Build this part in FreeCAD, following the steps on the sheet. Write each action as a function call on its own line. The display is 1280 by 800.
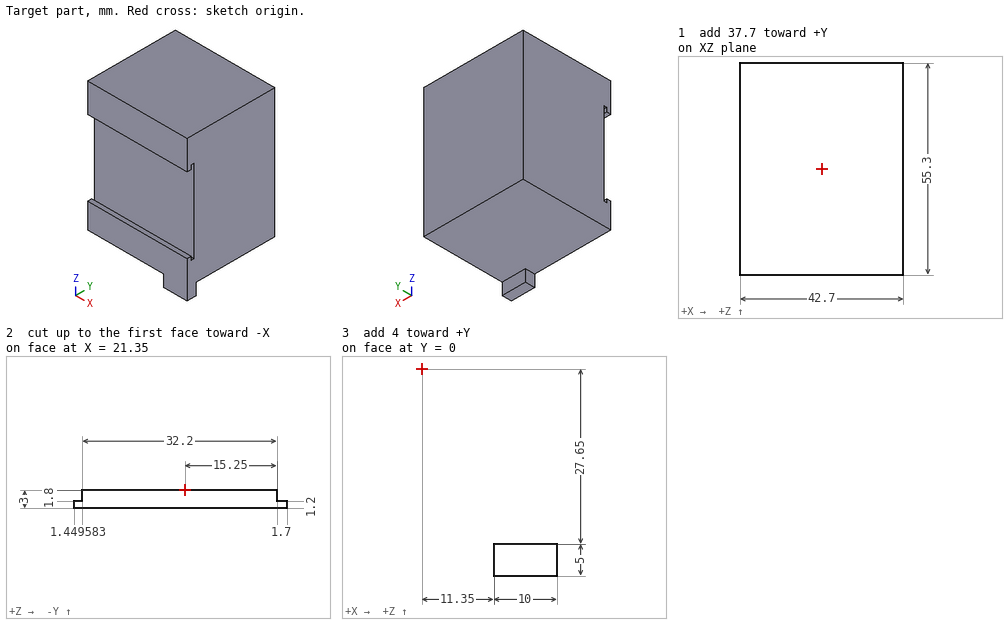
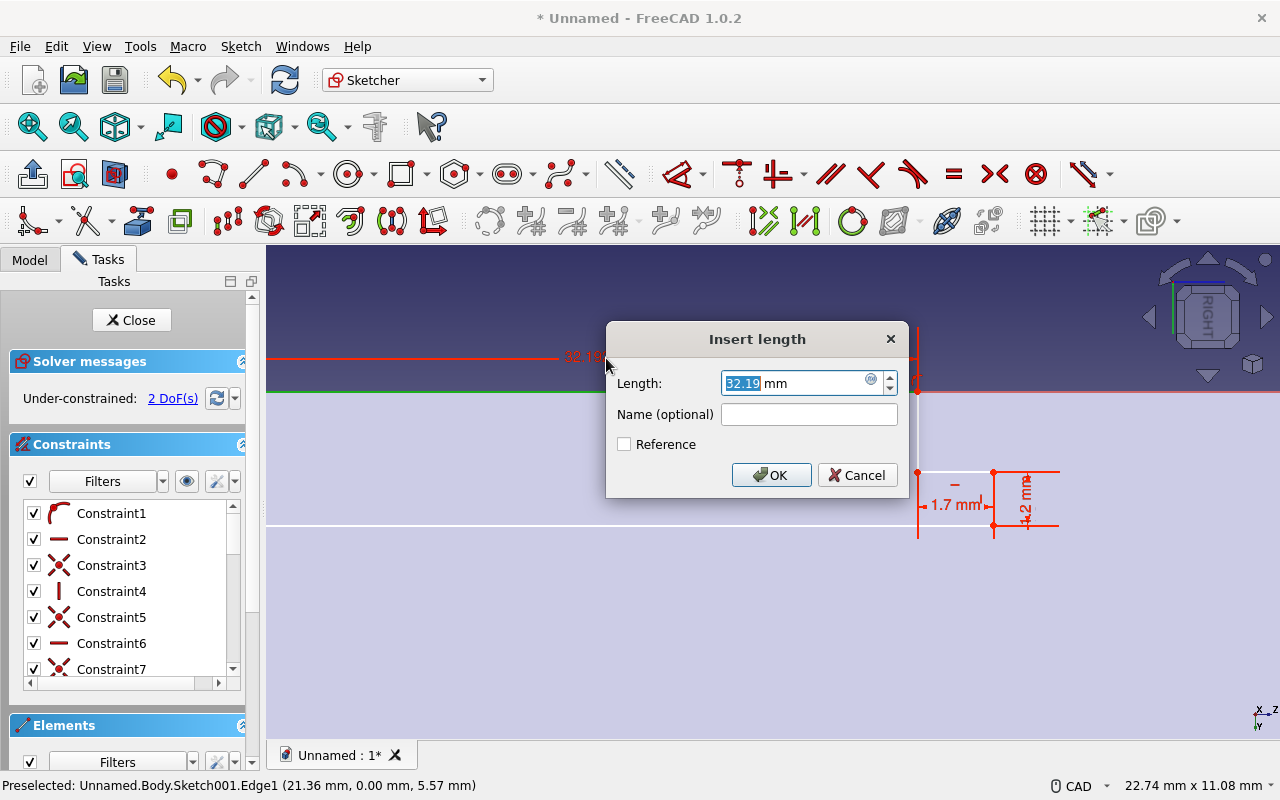
text(32.2)
key(Return)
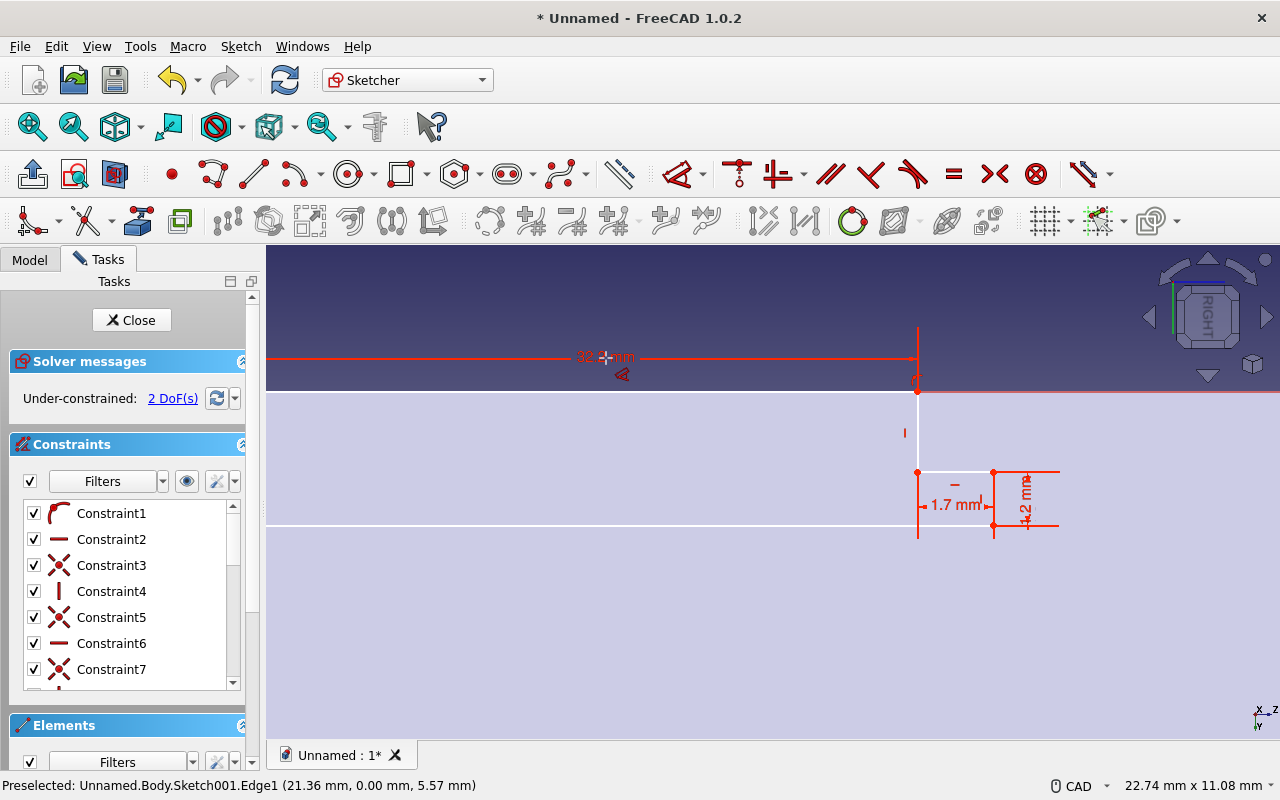
click(918, 392)
click(462, 358)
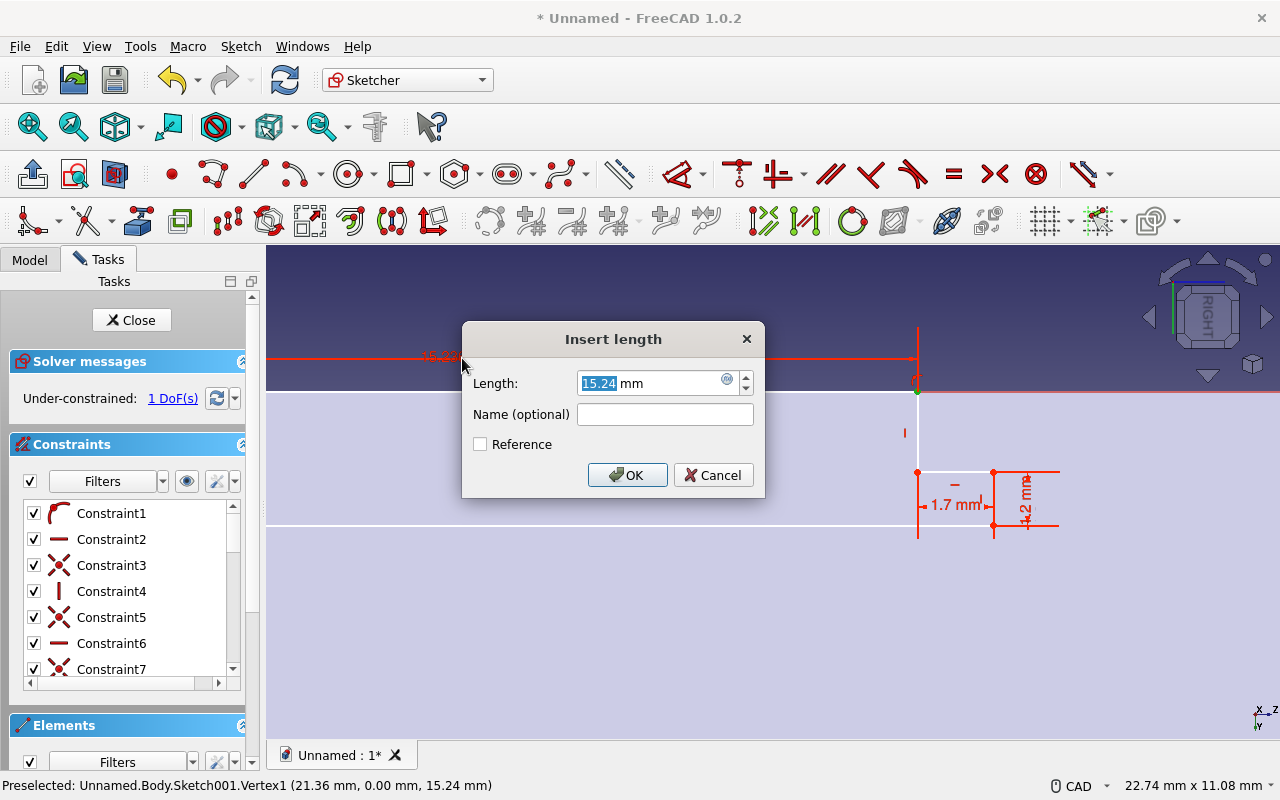
text(15.25)
key(Return)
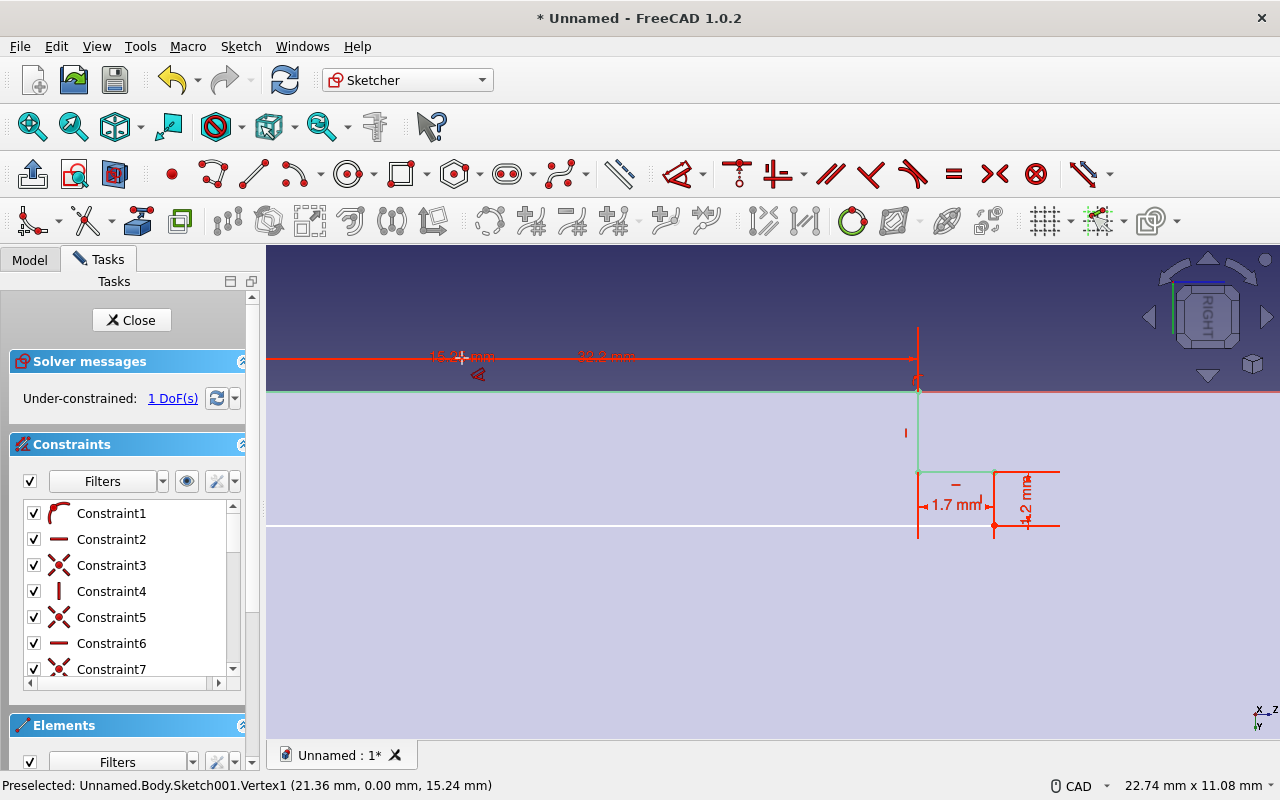
scroll(994, 511, down, 5)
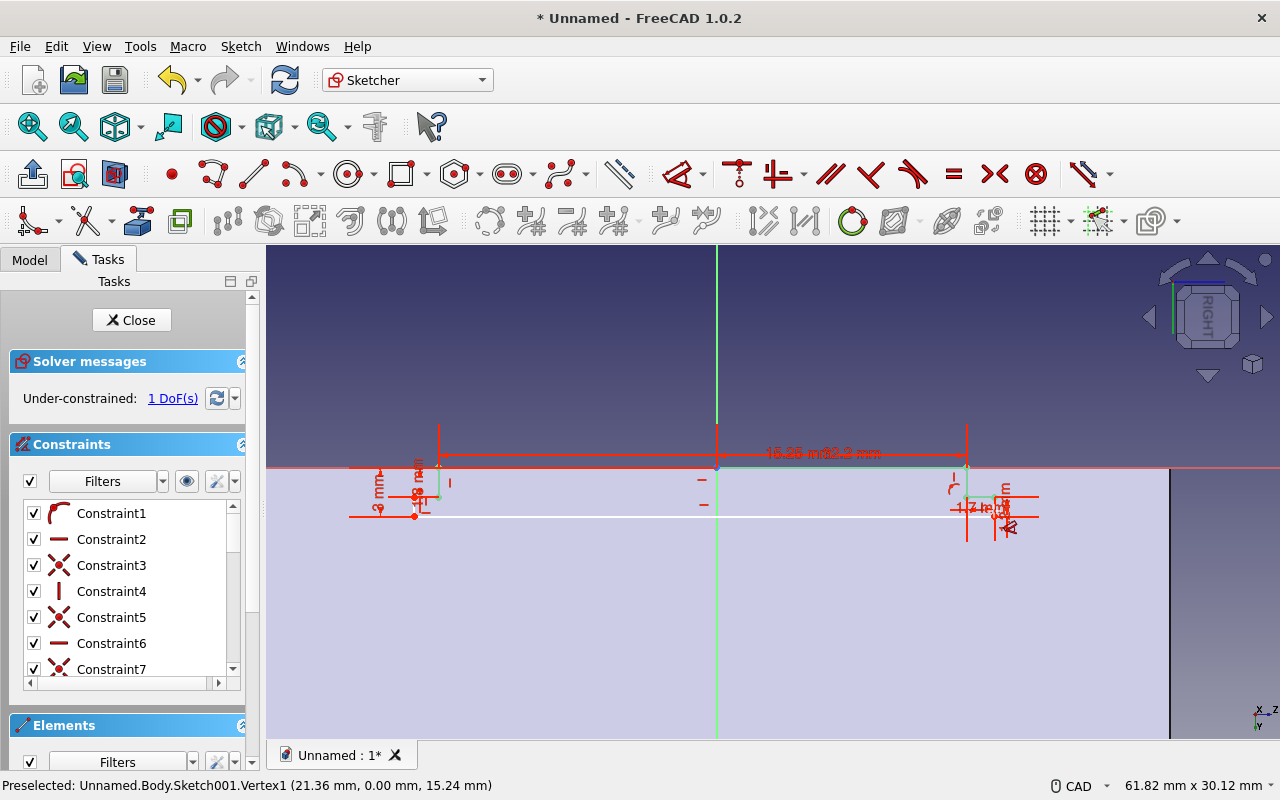
scroll(431, 497, up, 4)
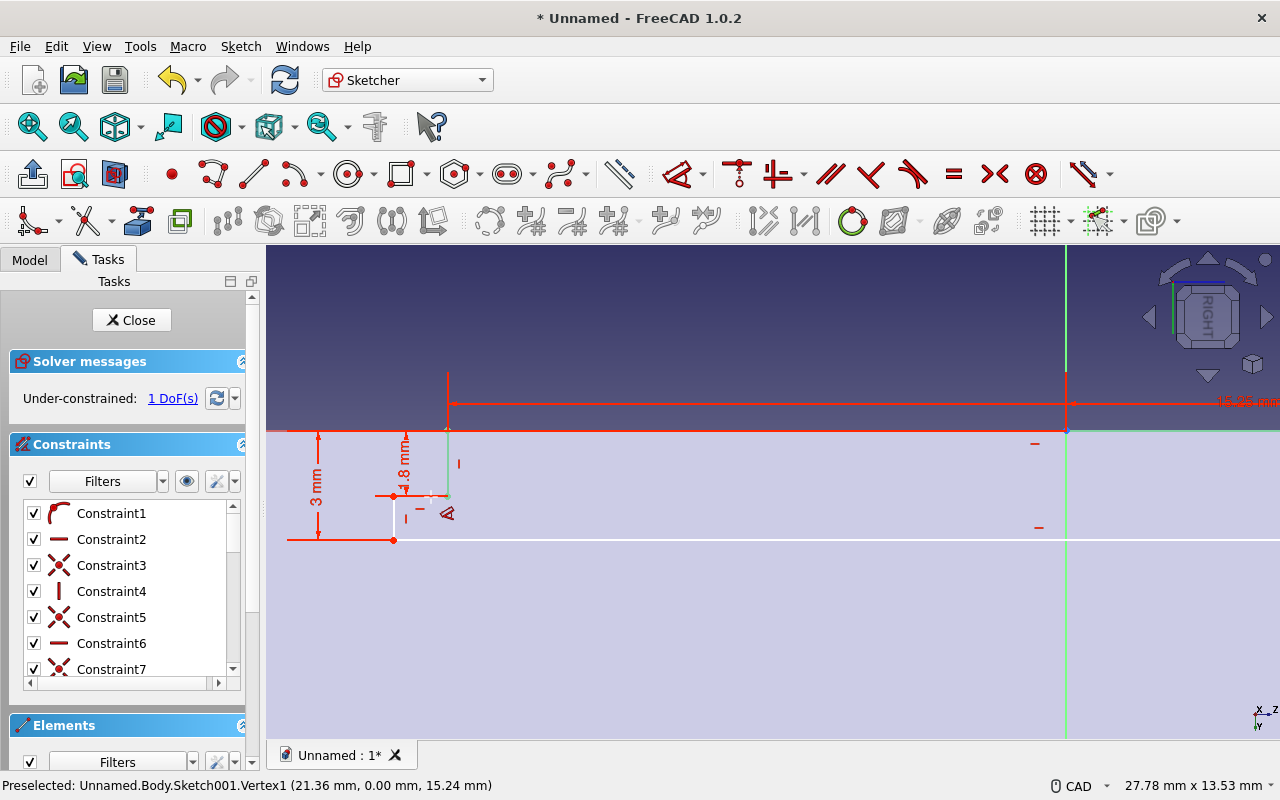
click(432, 496)
click(421, 554)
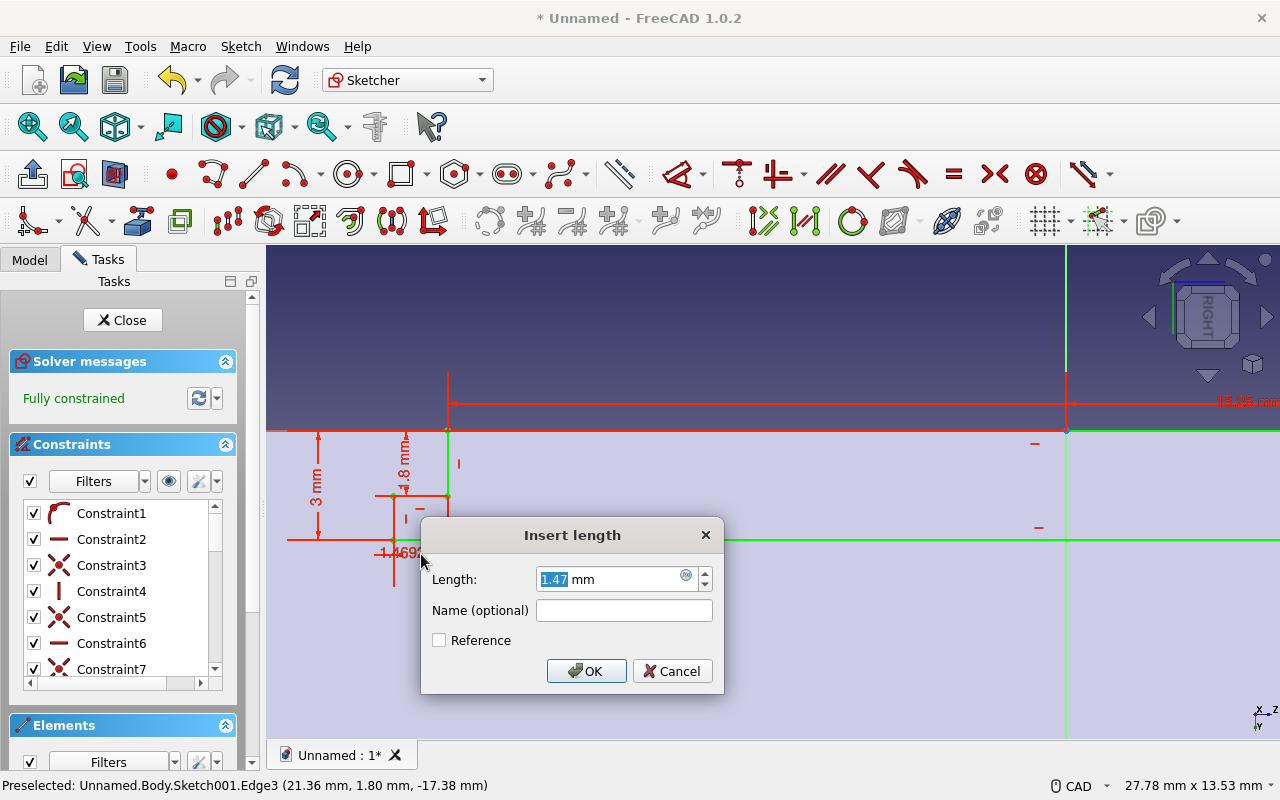
text(1.449583)
key(Return)
key(Escape)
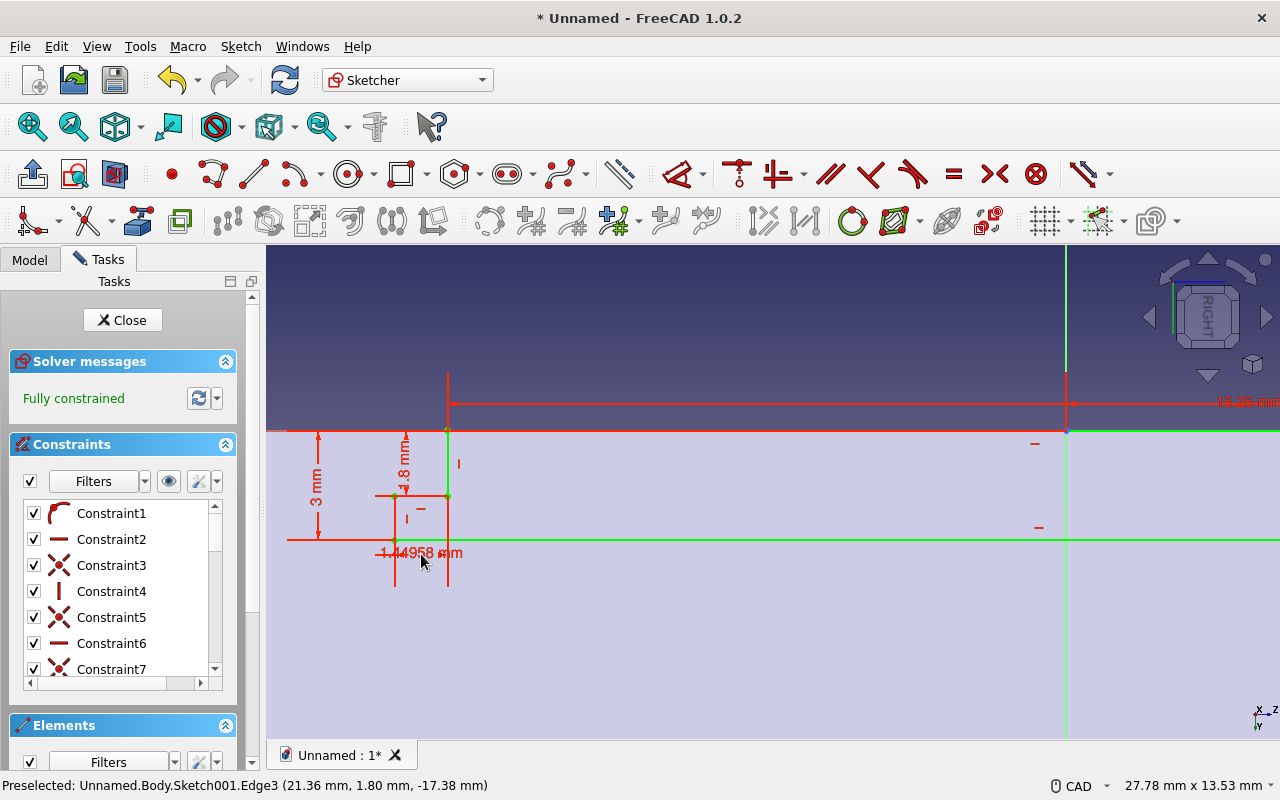
click(123, 320)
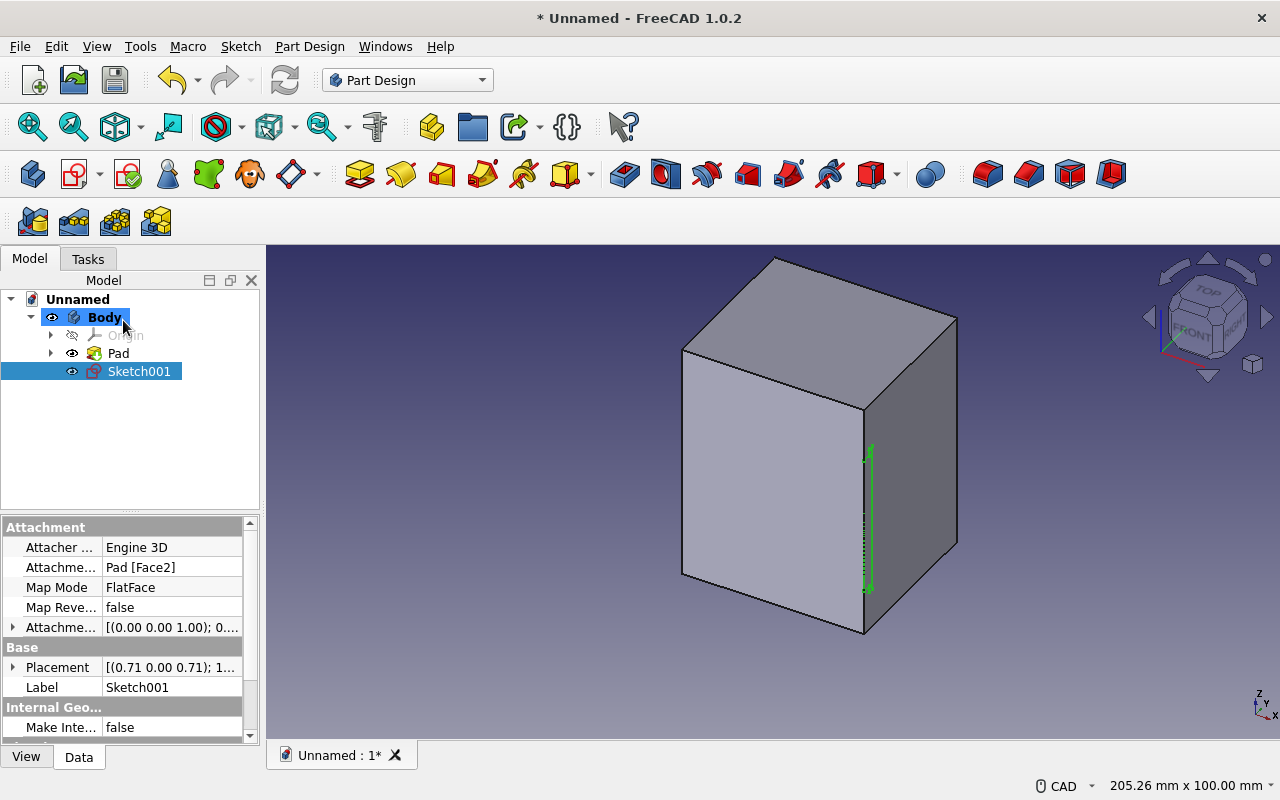
click(625, 174)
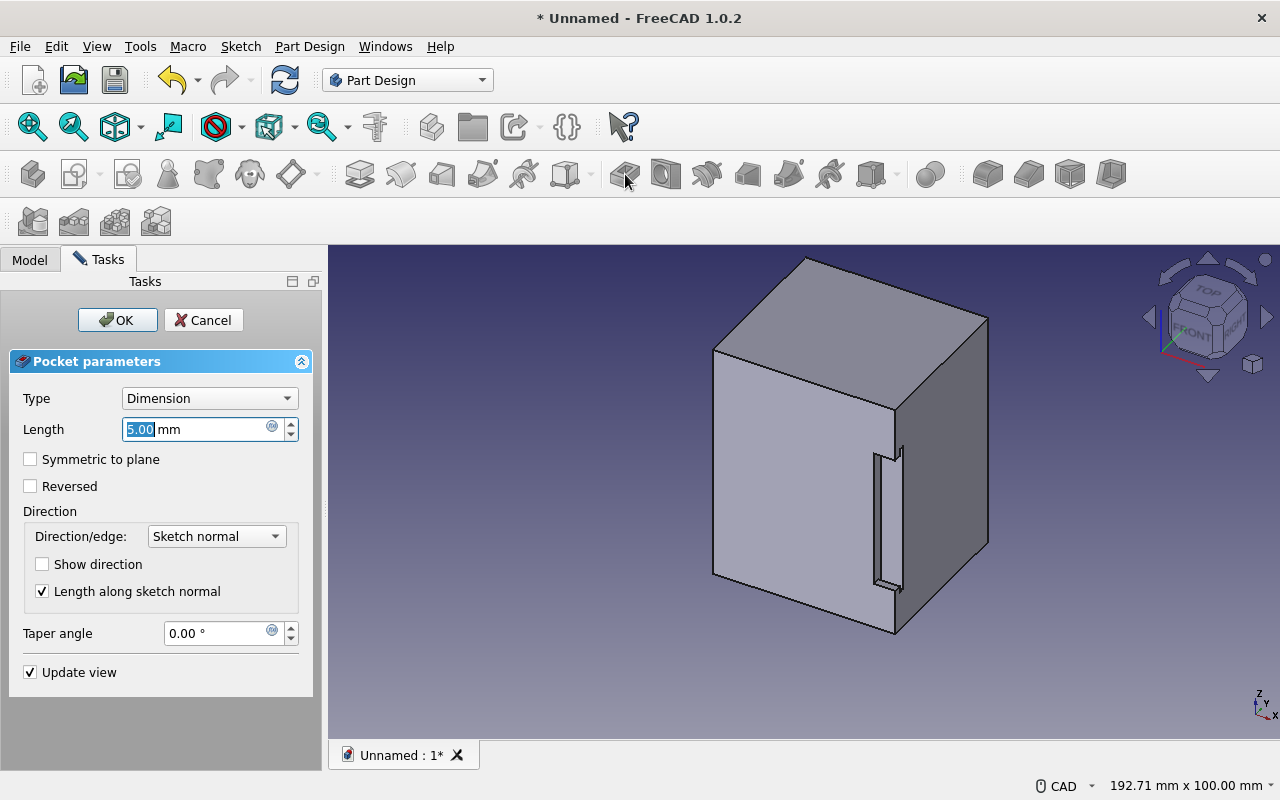
click(210, 398)